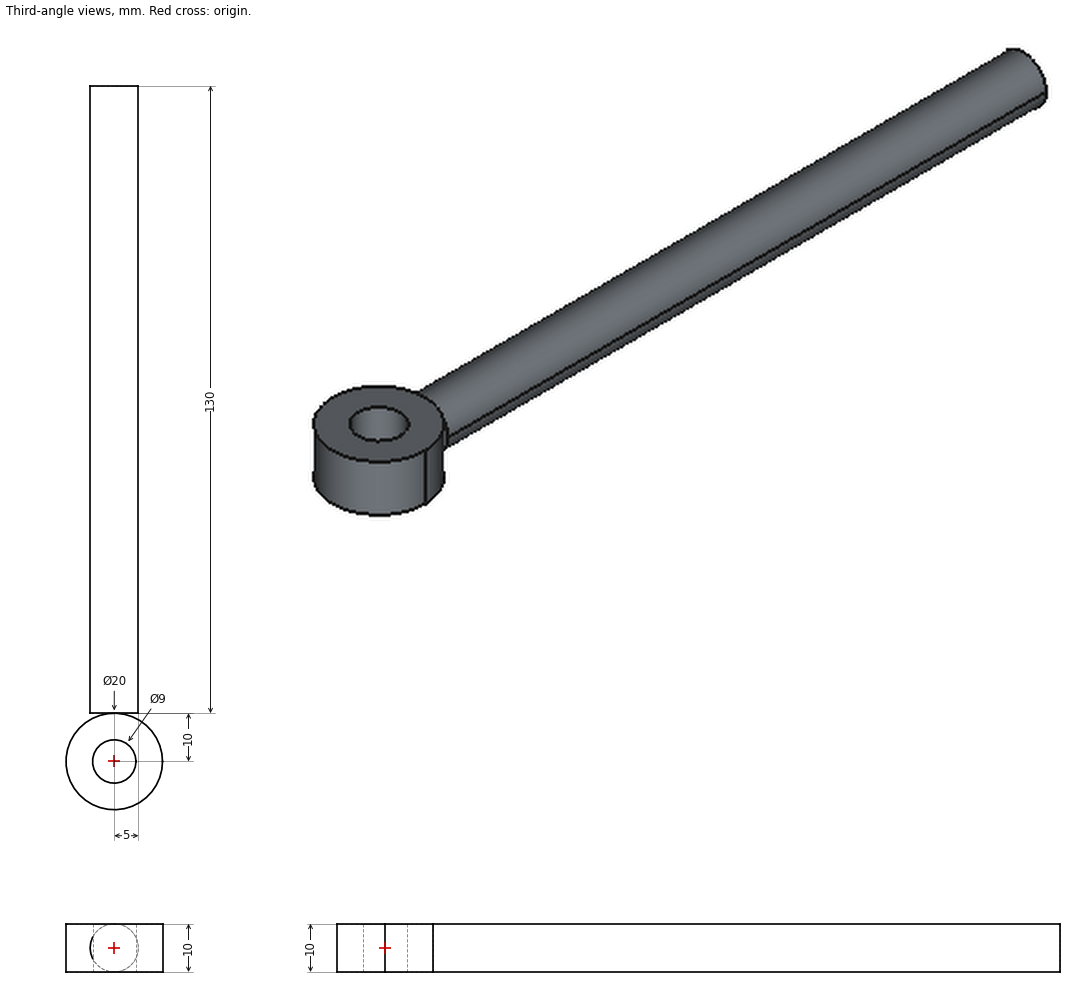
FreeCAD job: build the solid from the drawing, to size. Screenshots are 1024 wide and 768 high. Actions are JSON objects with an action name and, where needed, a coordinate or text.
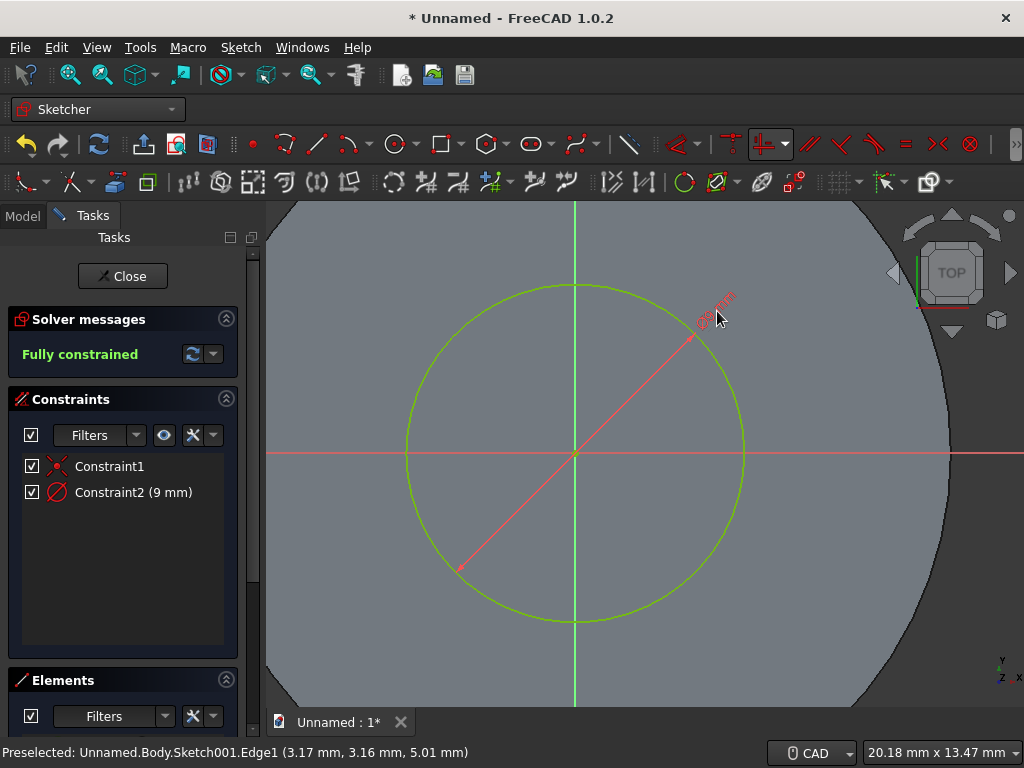
{"action": "left_click", "coordinate": [123, 276]}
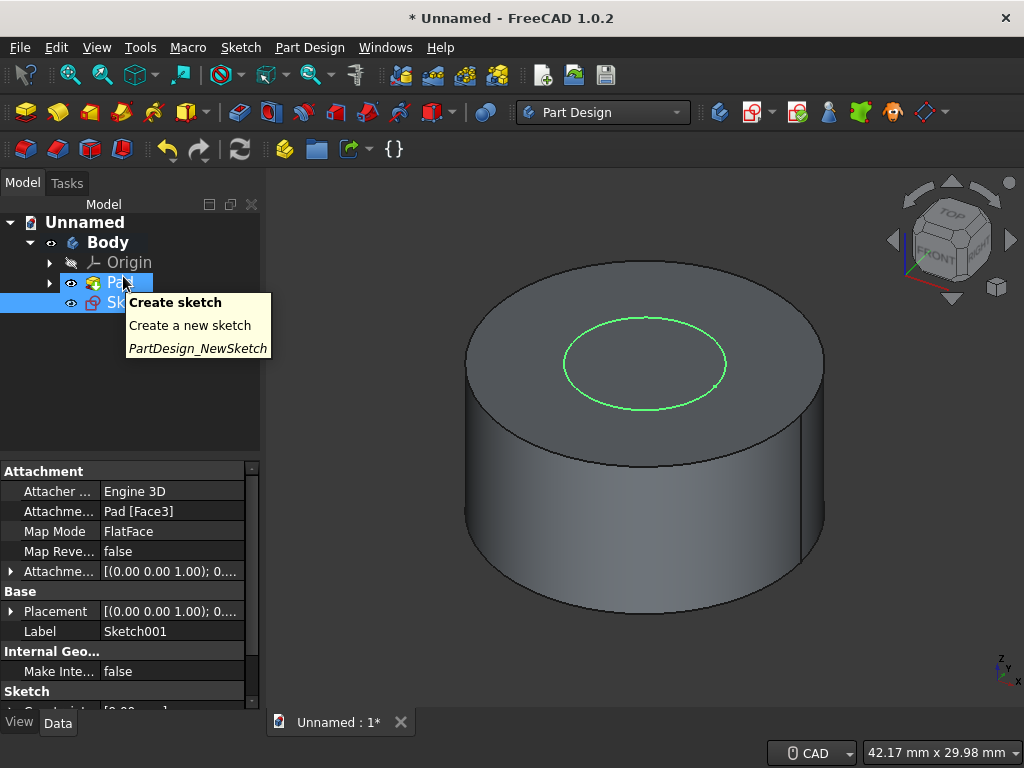
{"action": "left_click", "coordinate": [240, 112]}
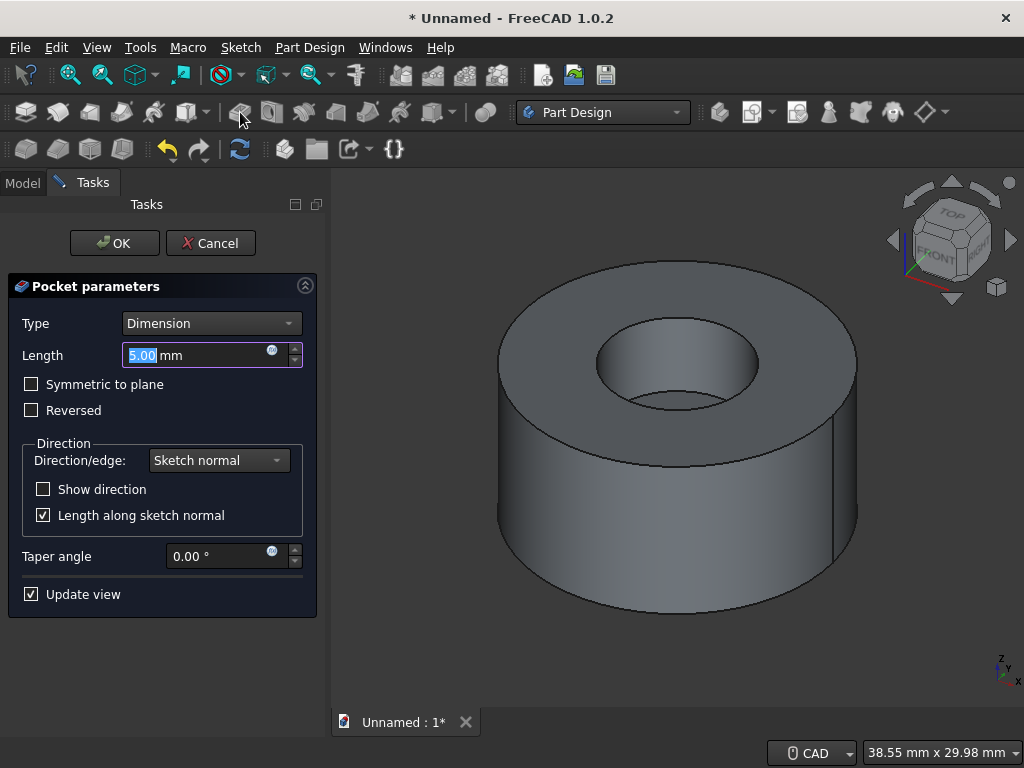
{"action": "type", "text": "10"}
{"action": "key", "text": "Tab"}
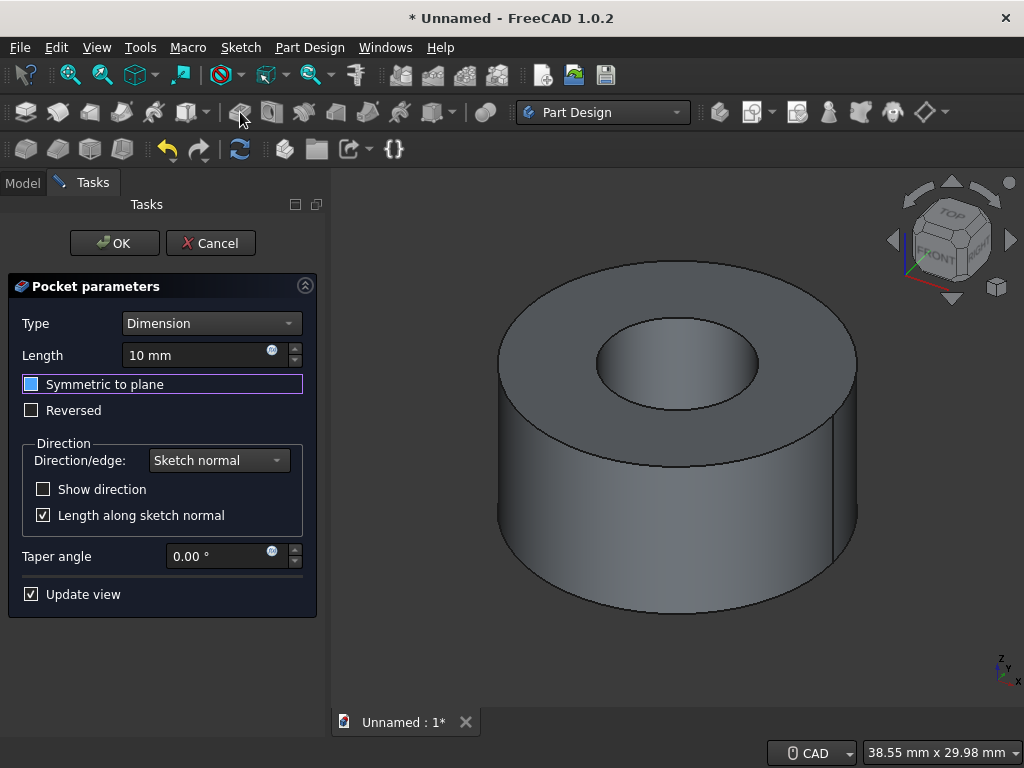
{"action": "left_click", "coordinate": [115, 243]}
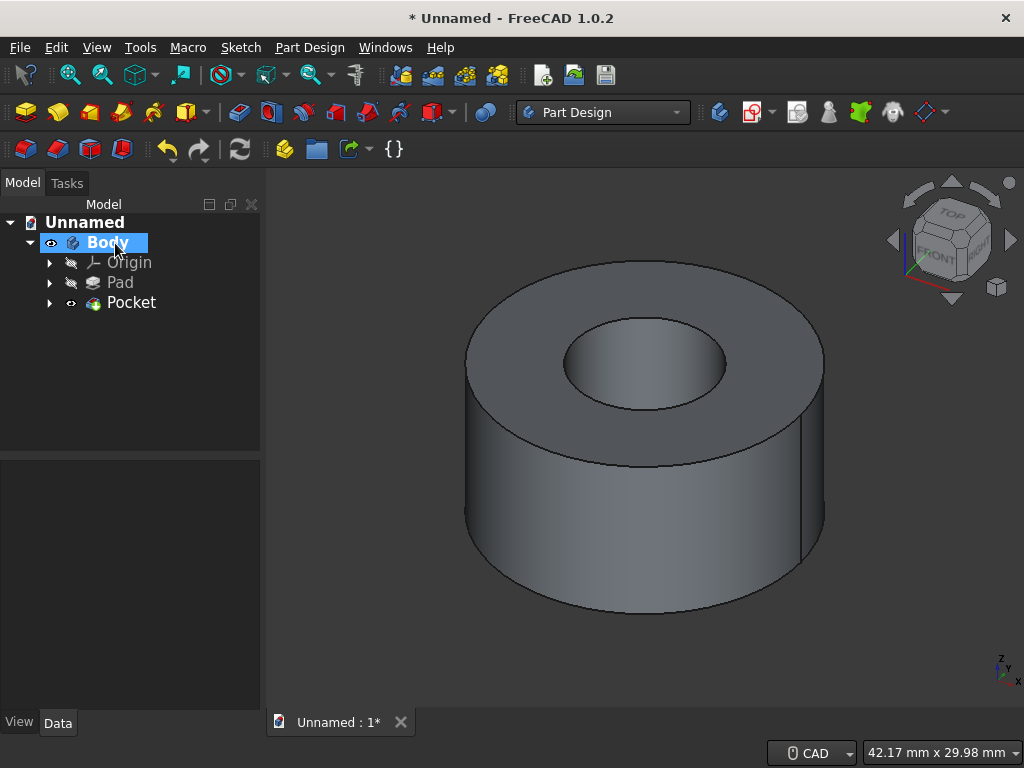
{"action": "left_click", "coordinate": [720, 112]}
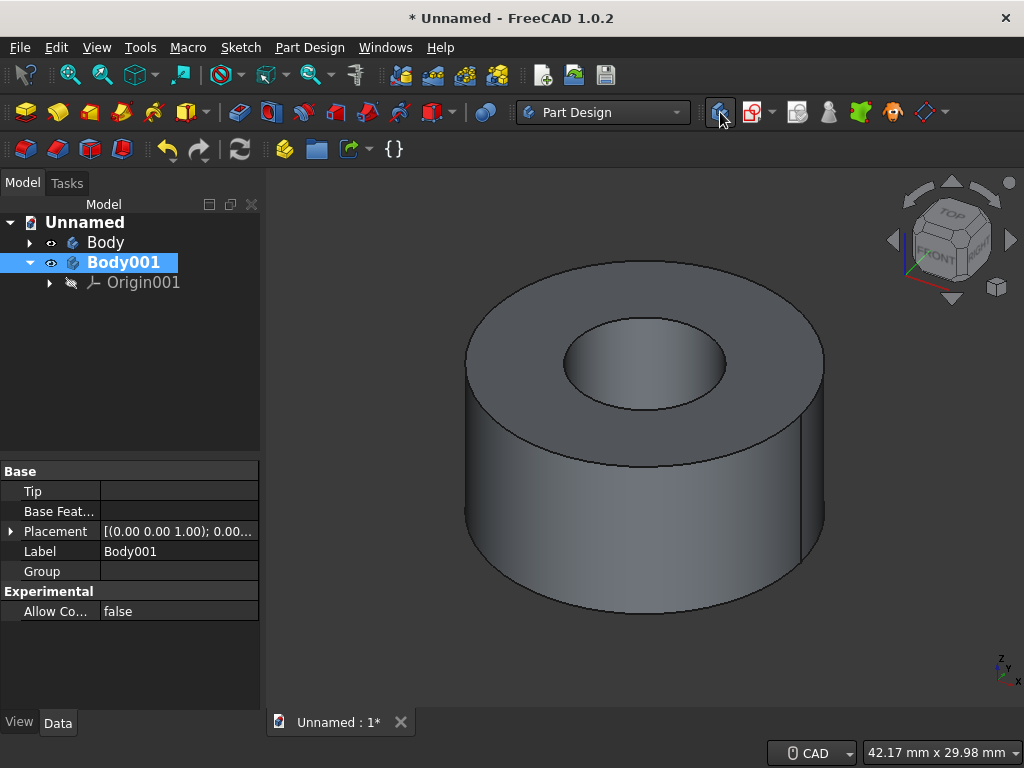
{"action": "left_click", "coordinate": [306, 667]}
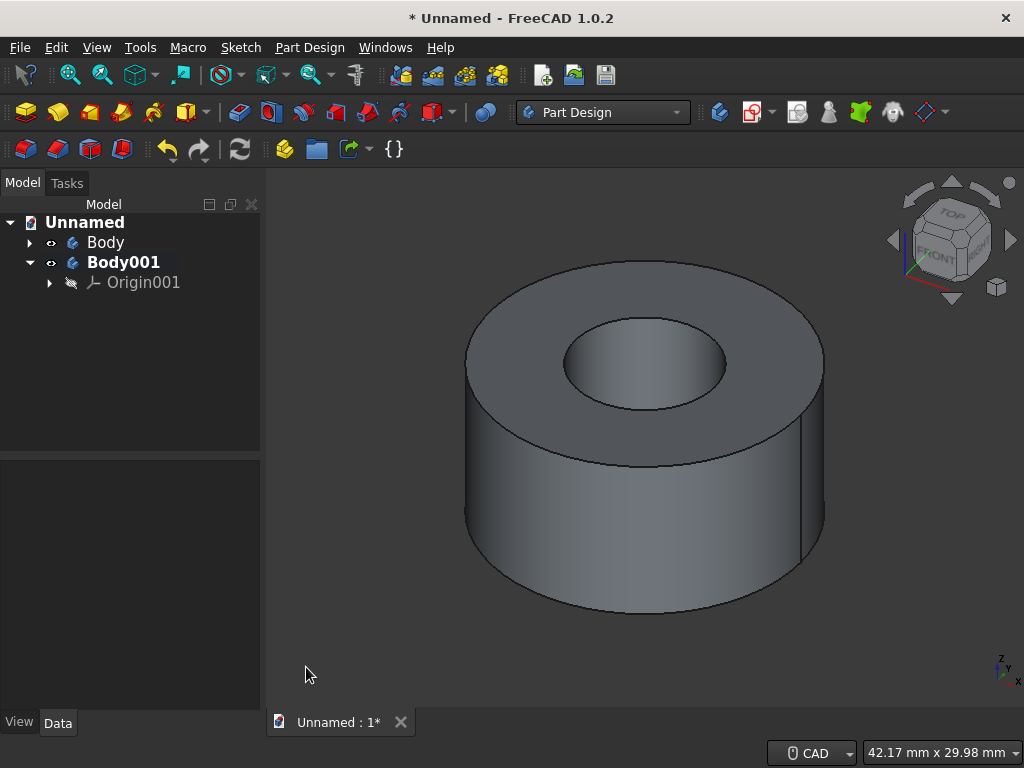
{"action": "left_click", "coordinate": [752, 112]}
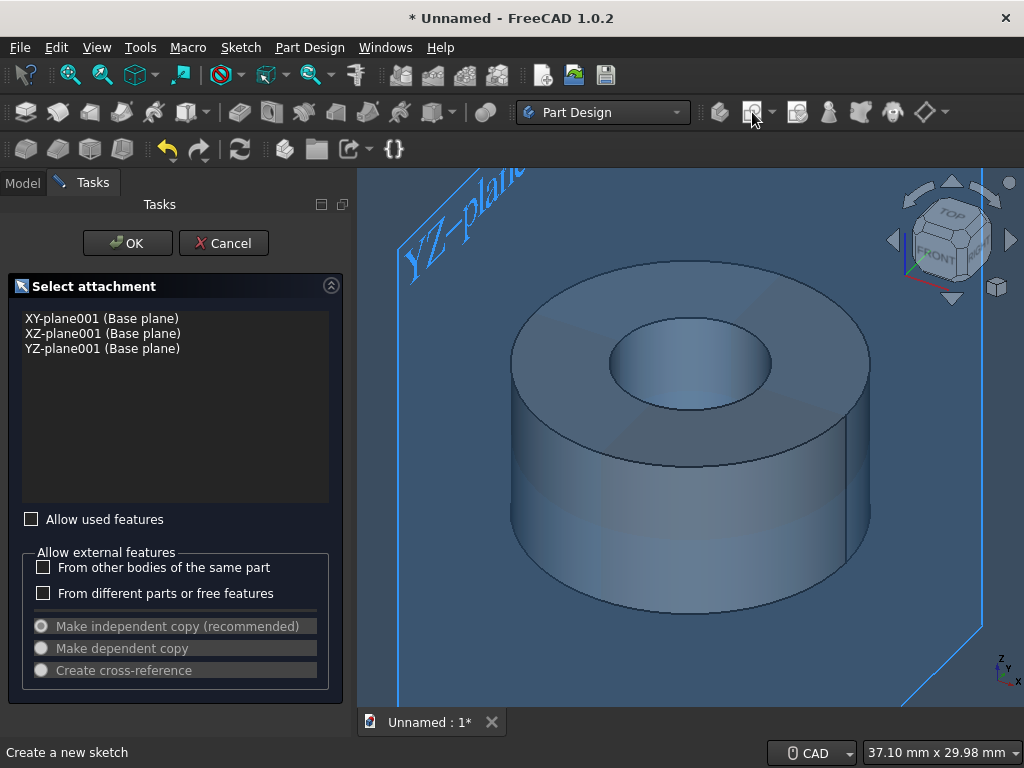
{"action": "left_click", "coordinate": [82, 318]}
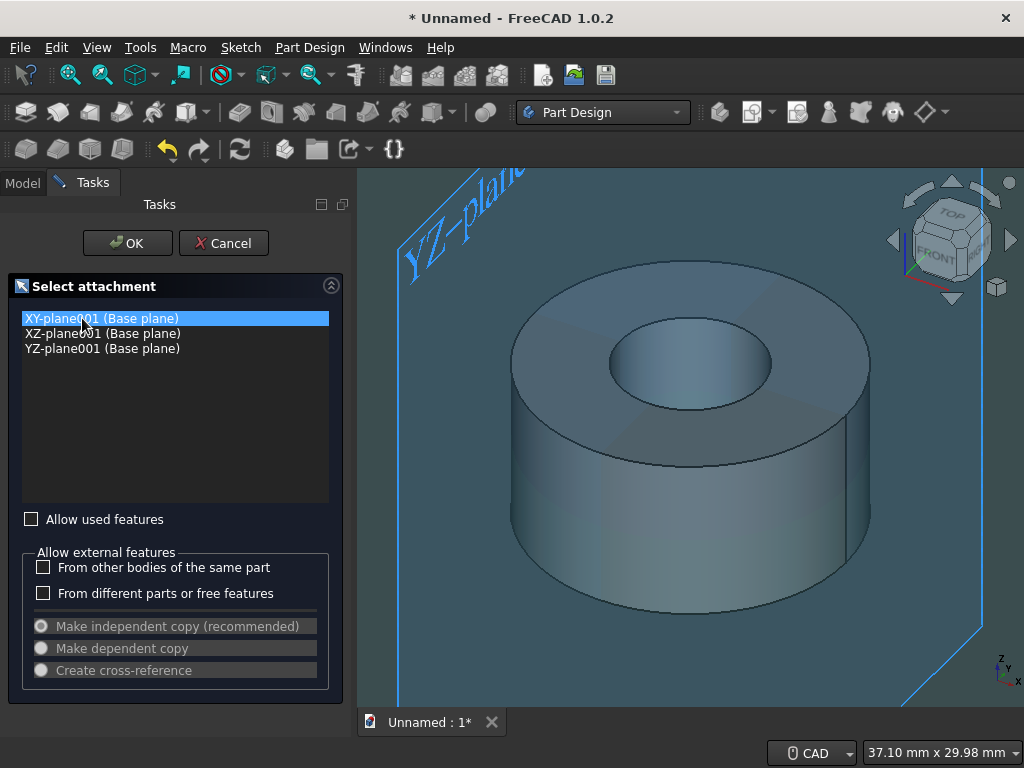
{"action": "left_click", "coordinate": [128, 243]}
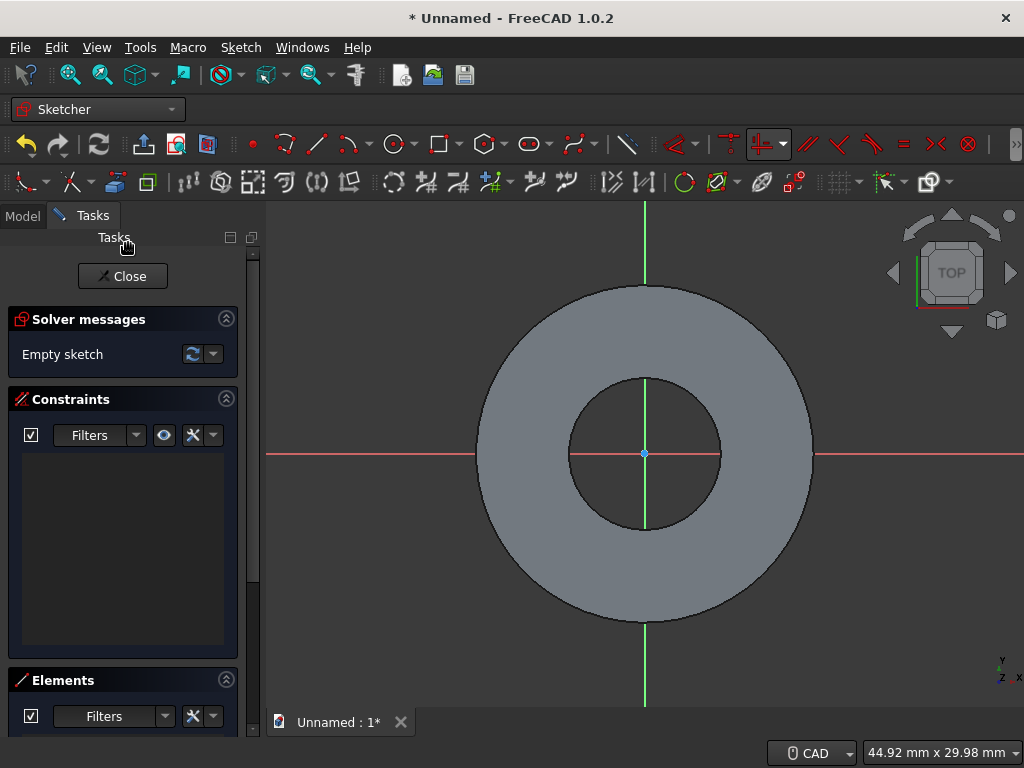
{"action": "scroll", "coordinate": [559, 639], "scroll_direction": "down", "scroll_amount": 10}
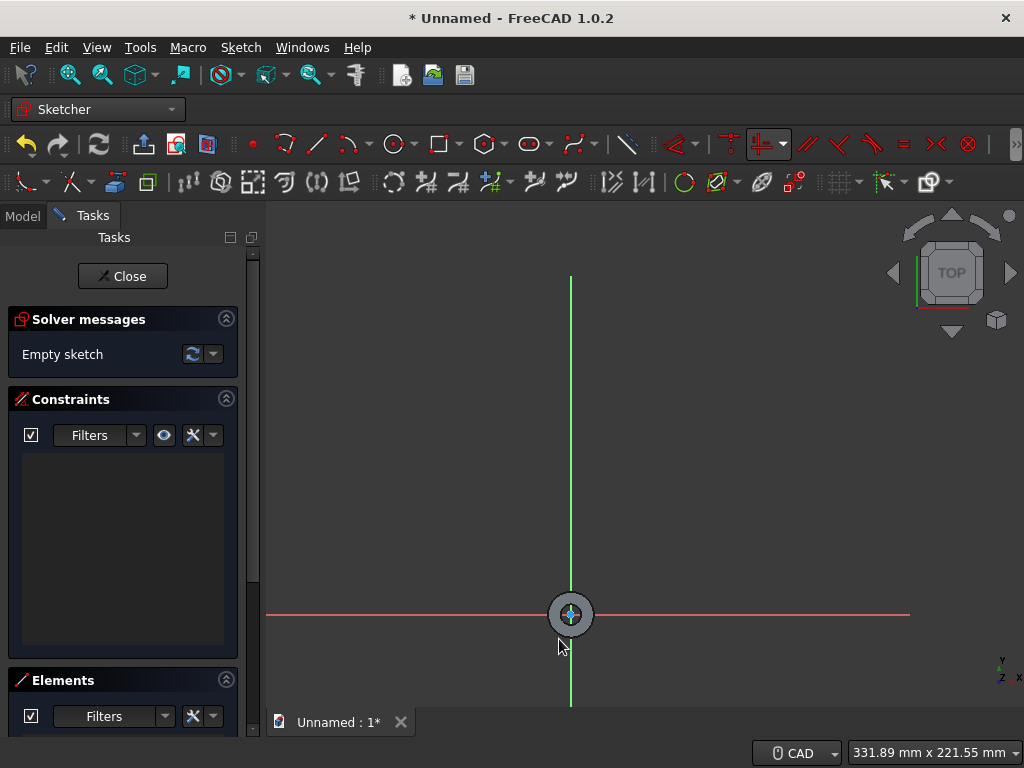
{"action": "left_click", "coordinate": [440, 144]}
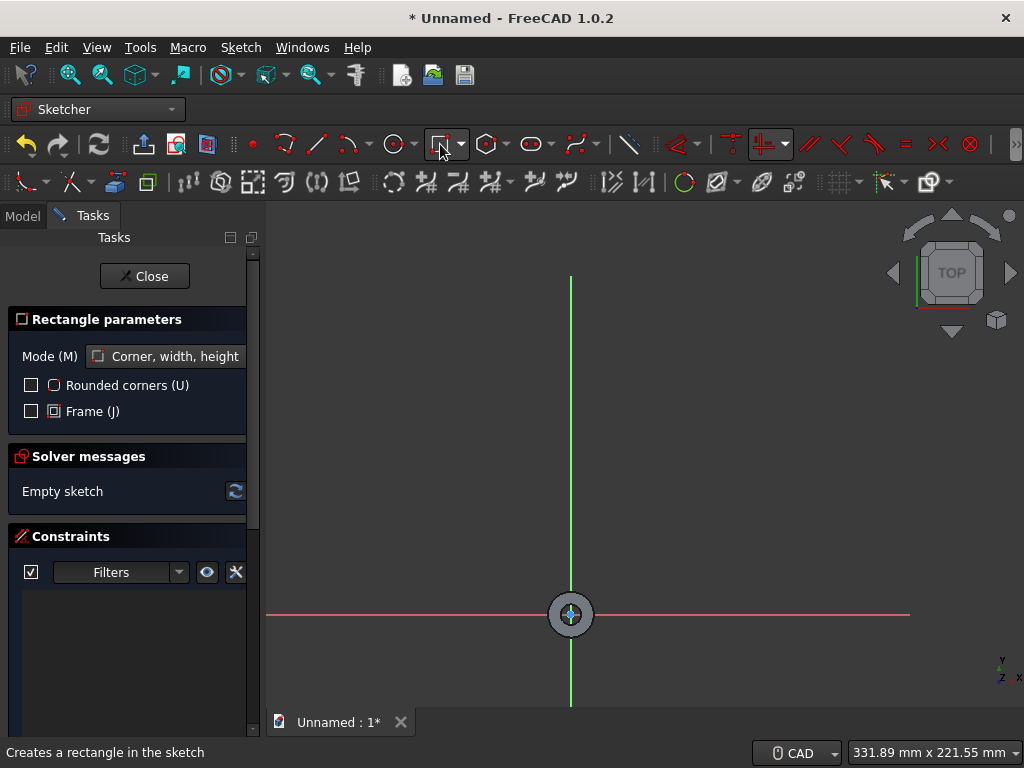
{"action": "scroll", "coordinate": [571, 295], "scroll_direction": "up", "scroll_amount": 2}